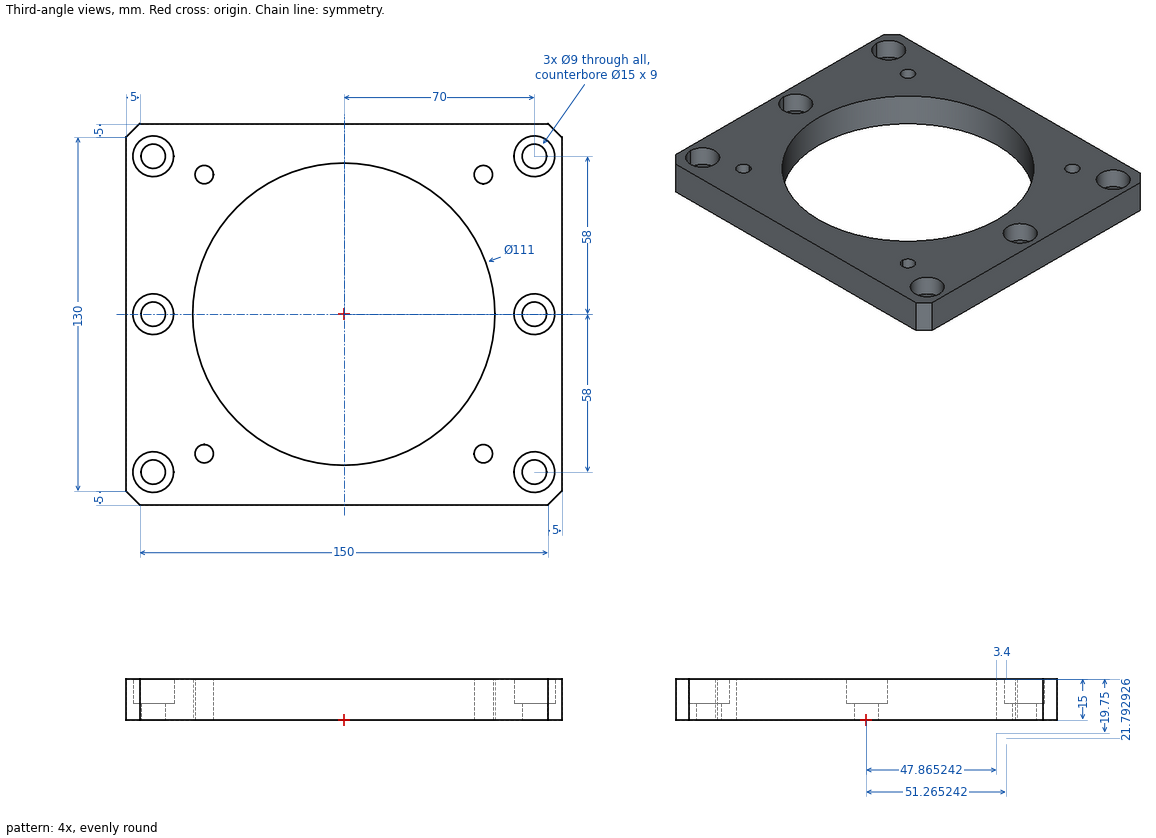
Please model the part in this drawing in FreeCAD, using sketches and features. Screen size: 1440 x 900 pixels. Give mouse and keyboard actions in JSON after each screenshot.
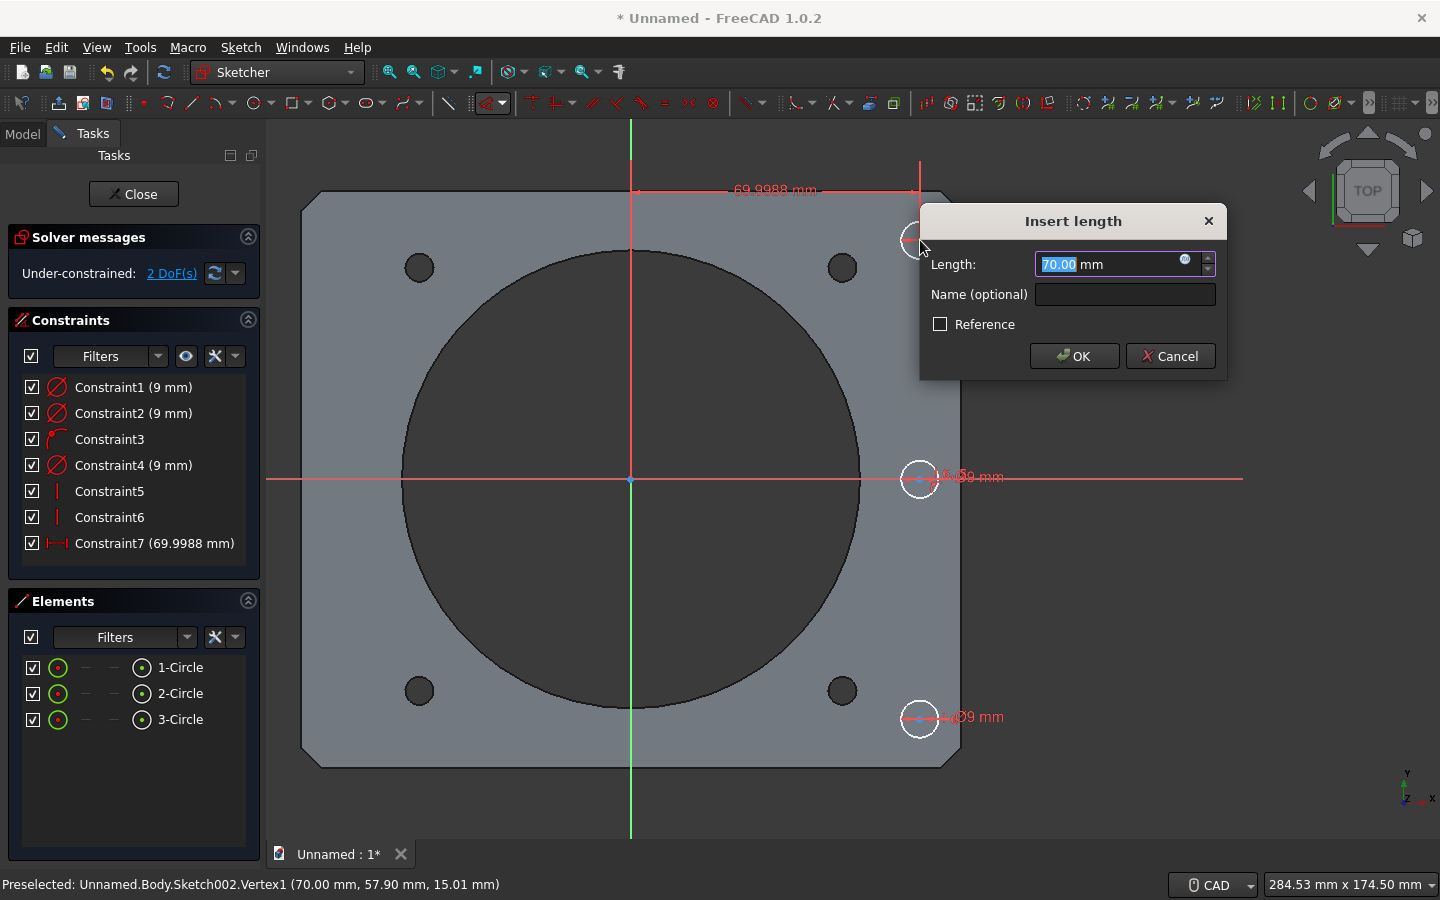
{"action": "type", "text": "70"}
{"action": "key", "text": "Return"}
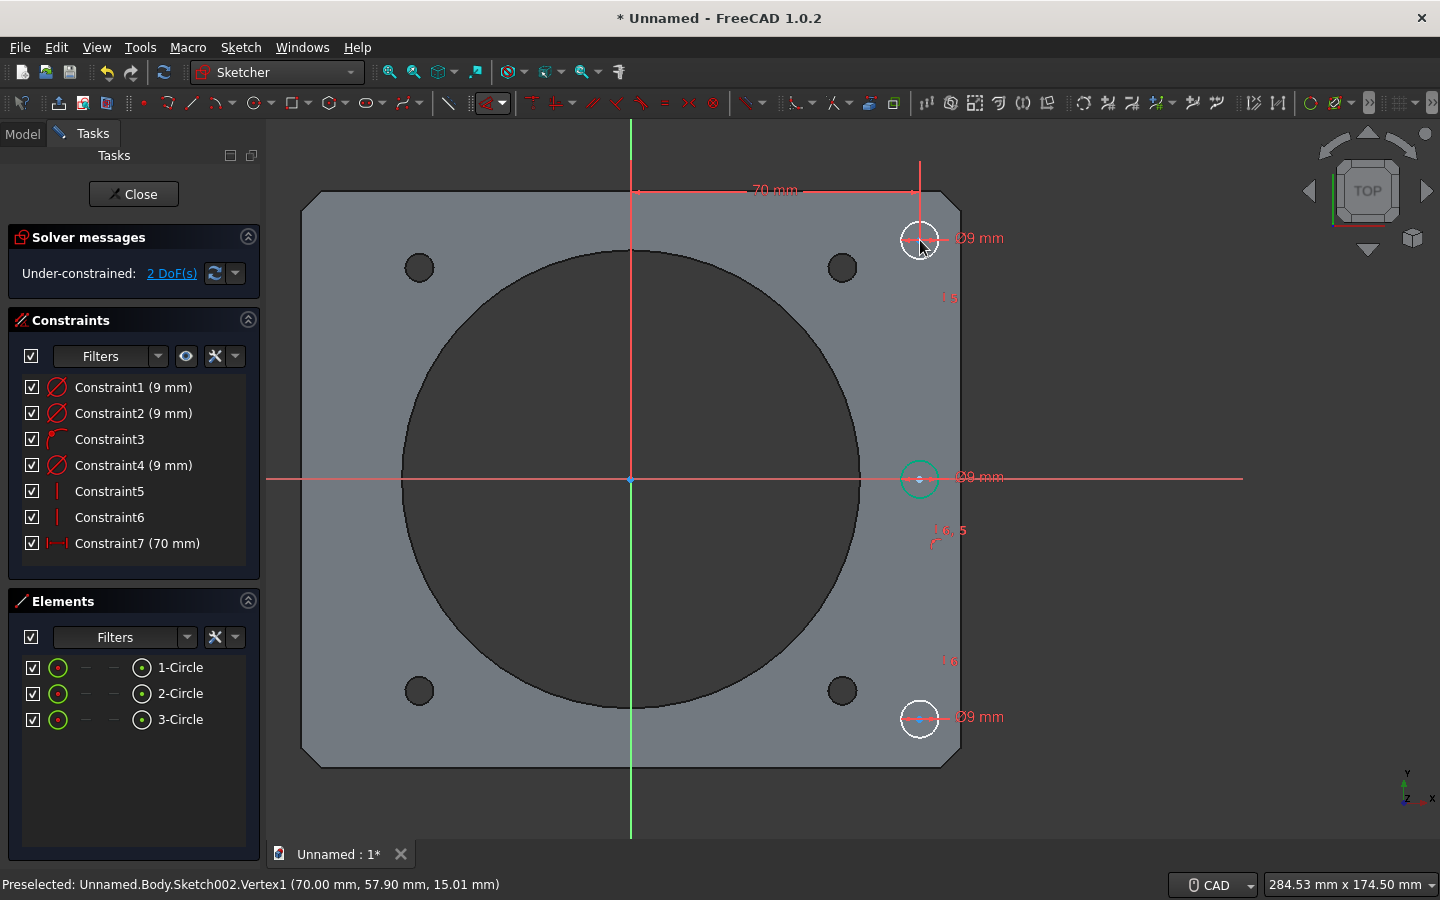
{"action": "left_click", "coordinate": [920, 240]}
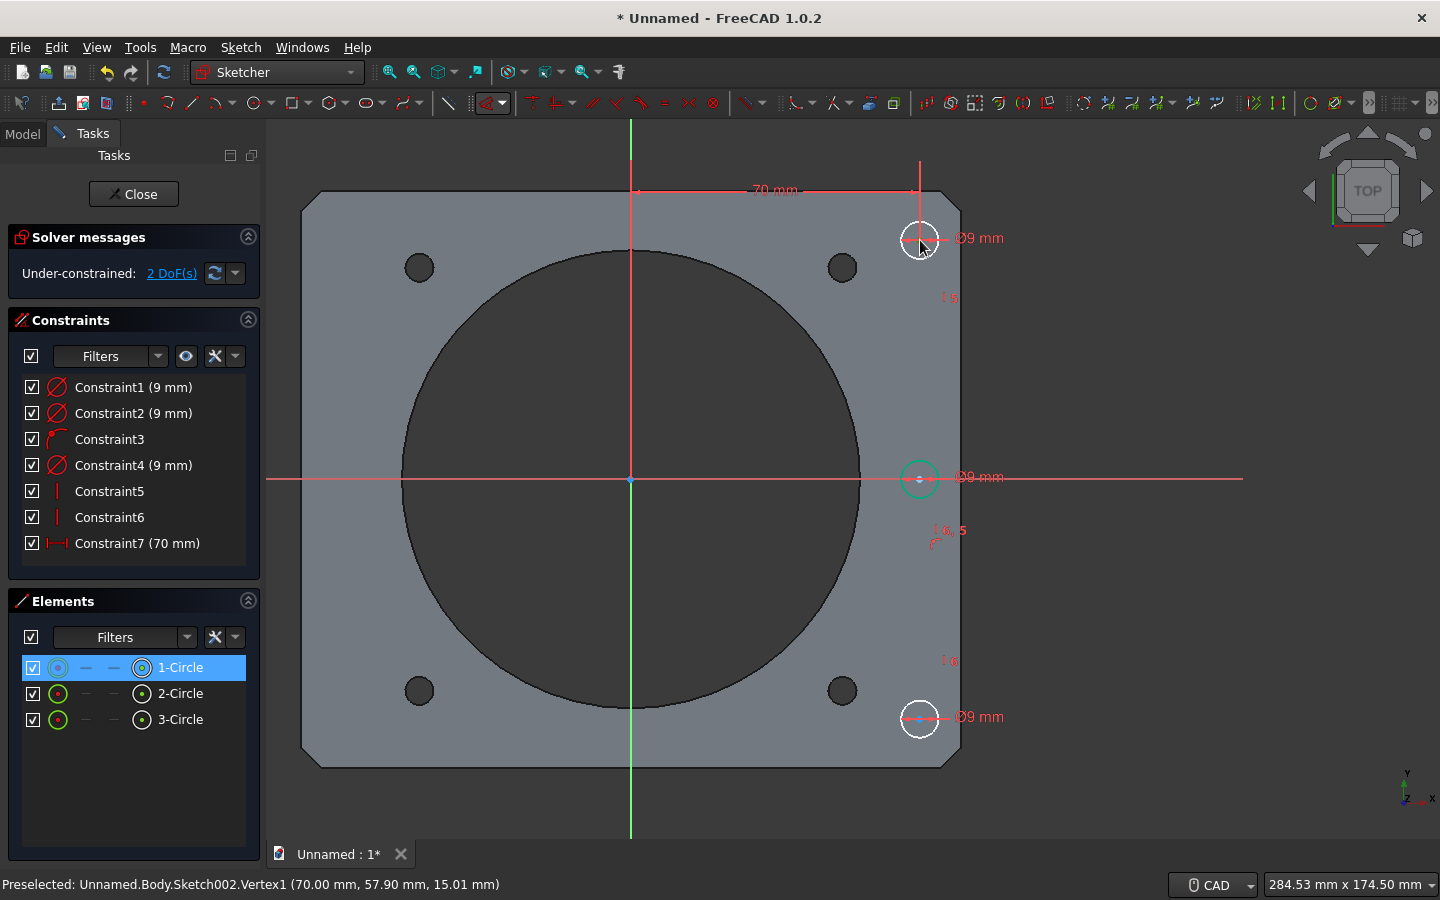
{"action": "left_click", "coordinate": [504, 104]}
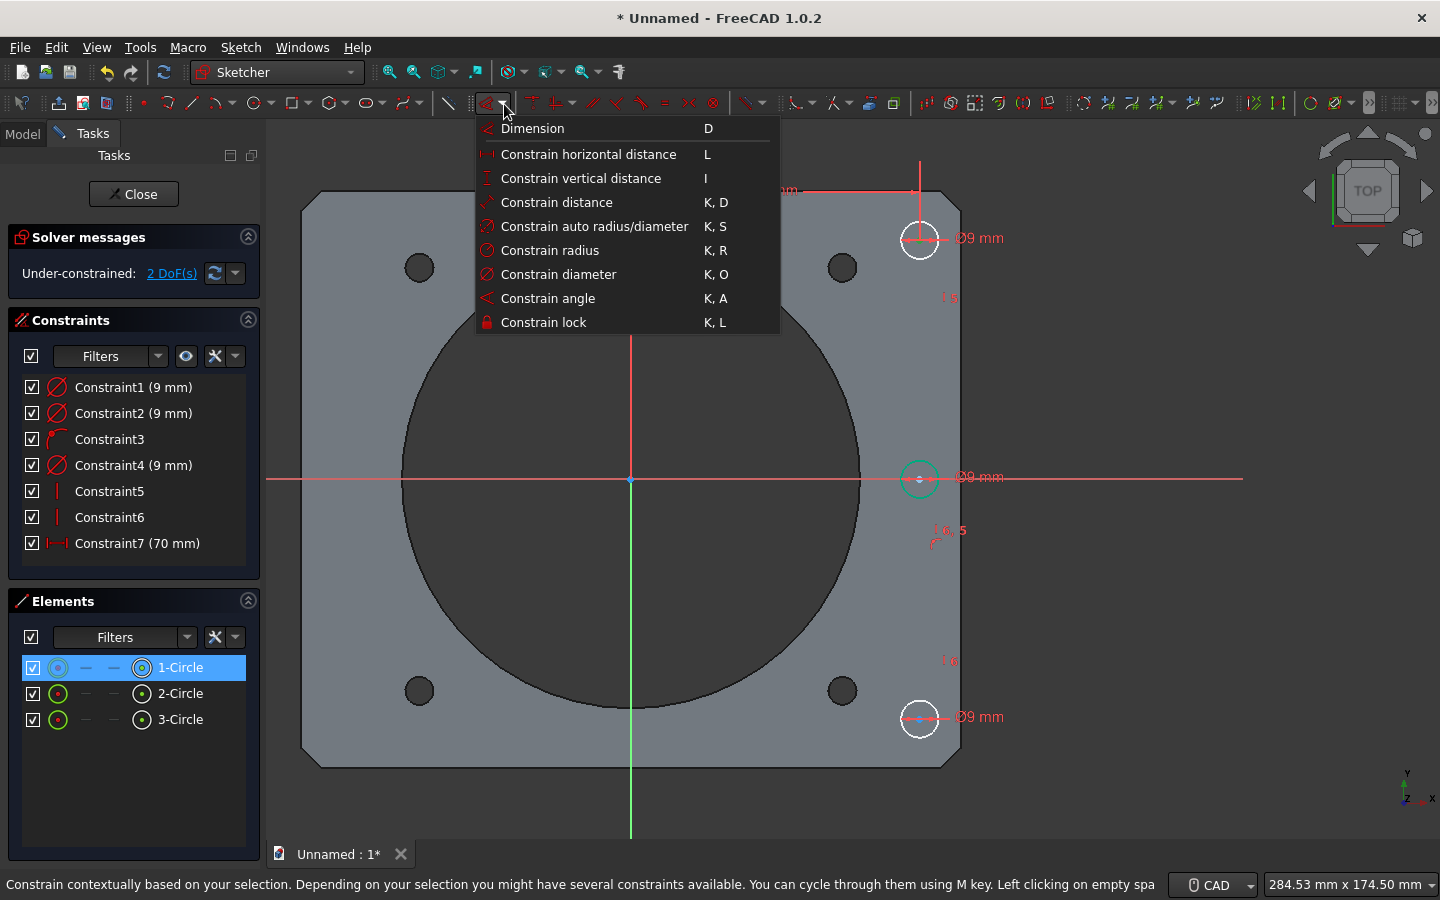
{"action": "left_click", "coordinate": [628, 178]}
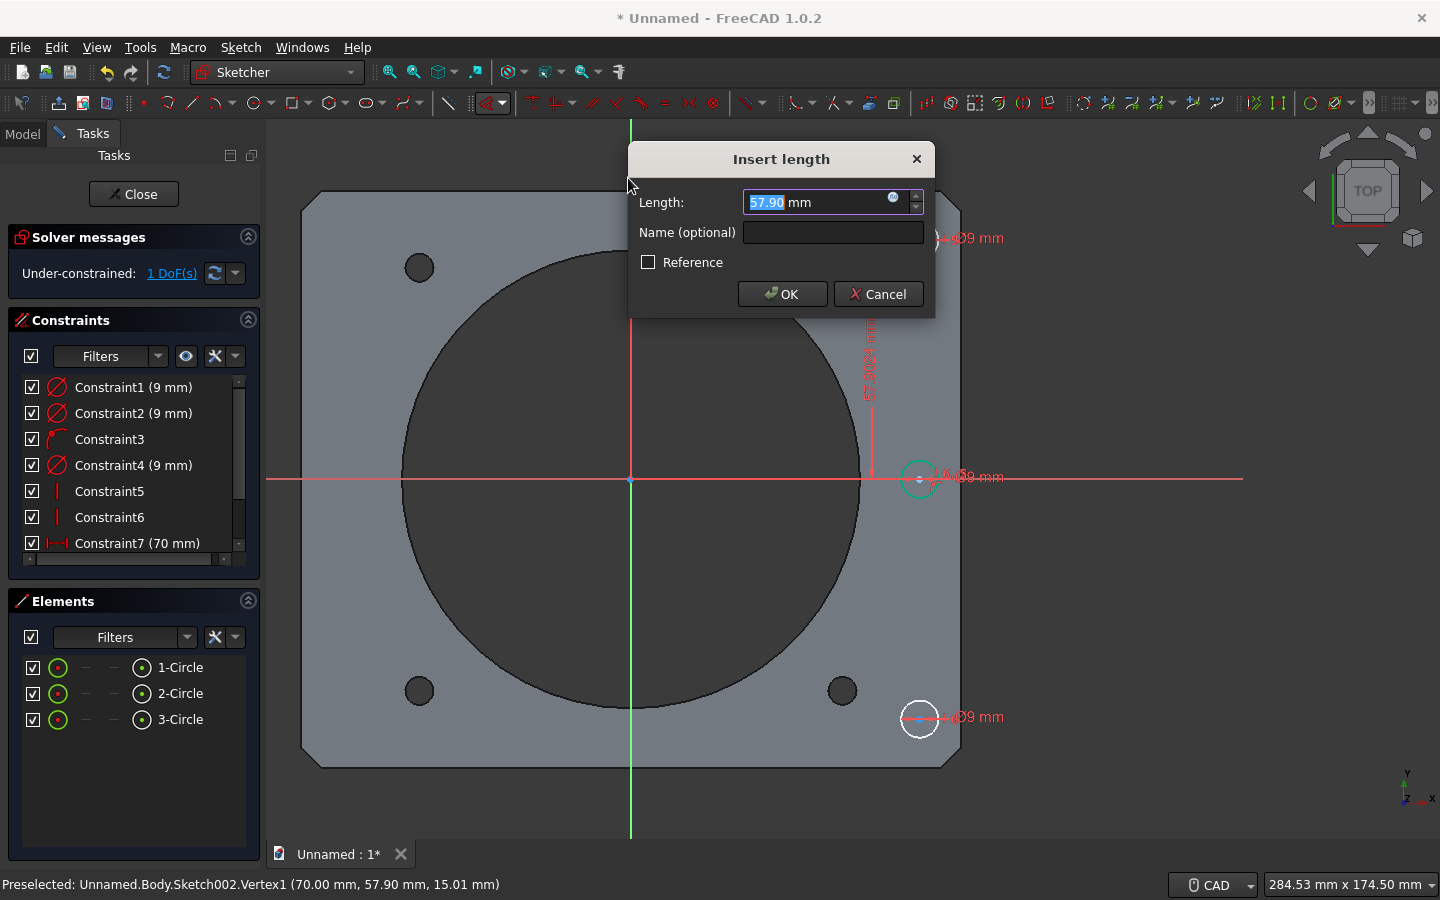
{"action": "type", "text": "58"}
{"action": "key", "text": "Return"}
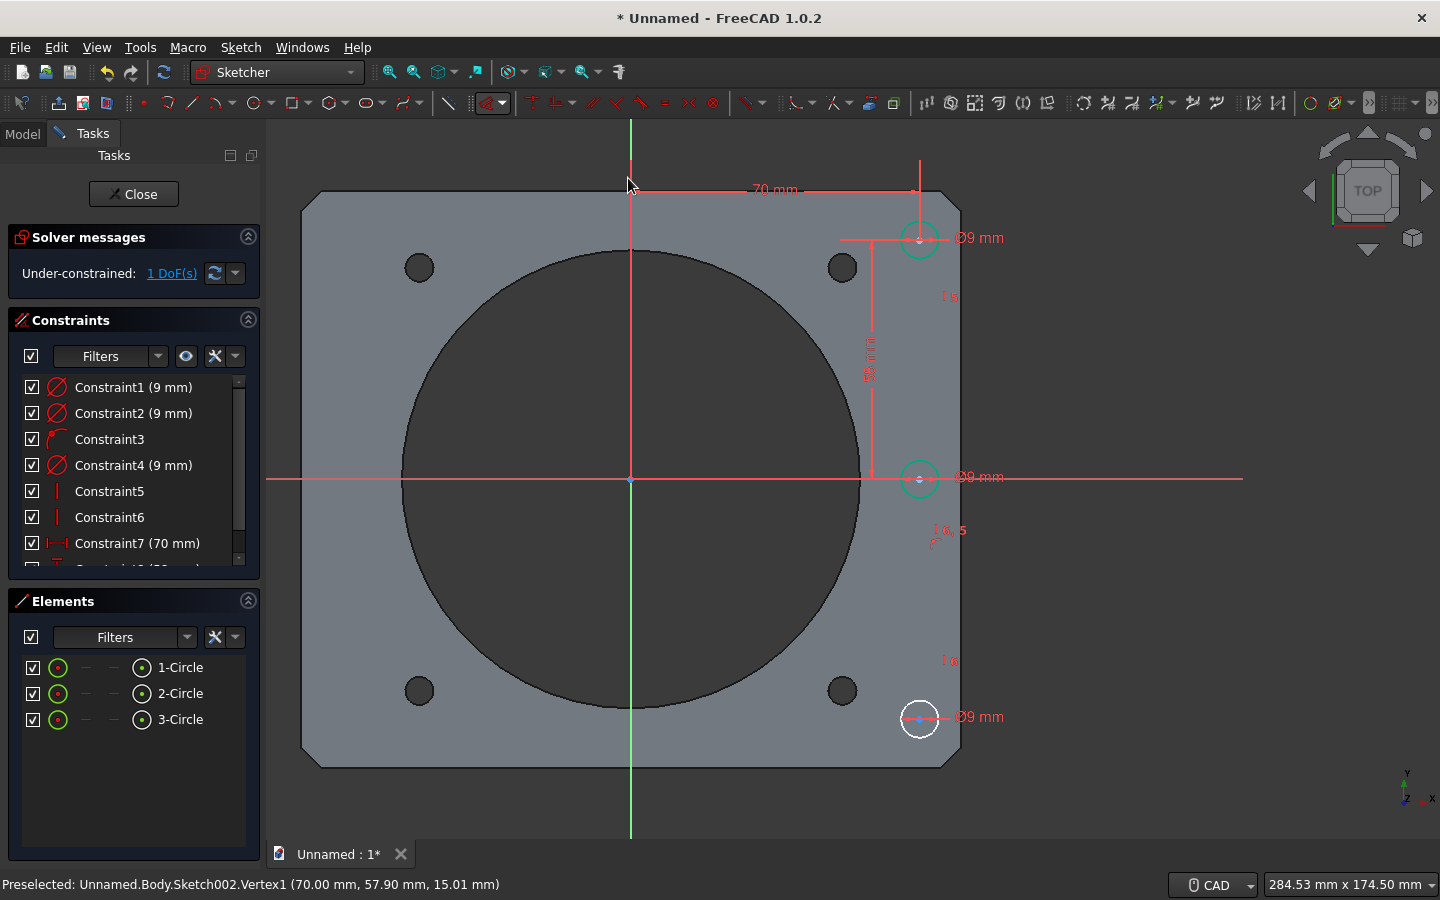
{"action": "left_click", "coordinate": [920, 719]}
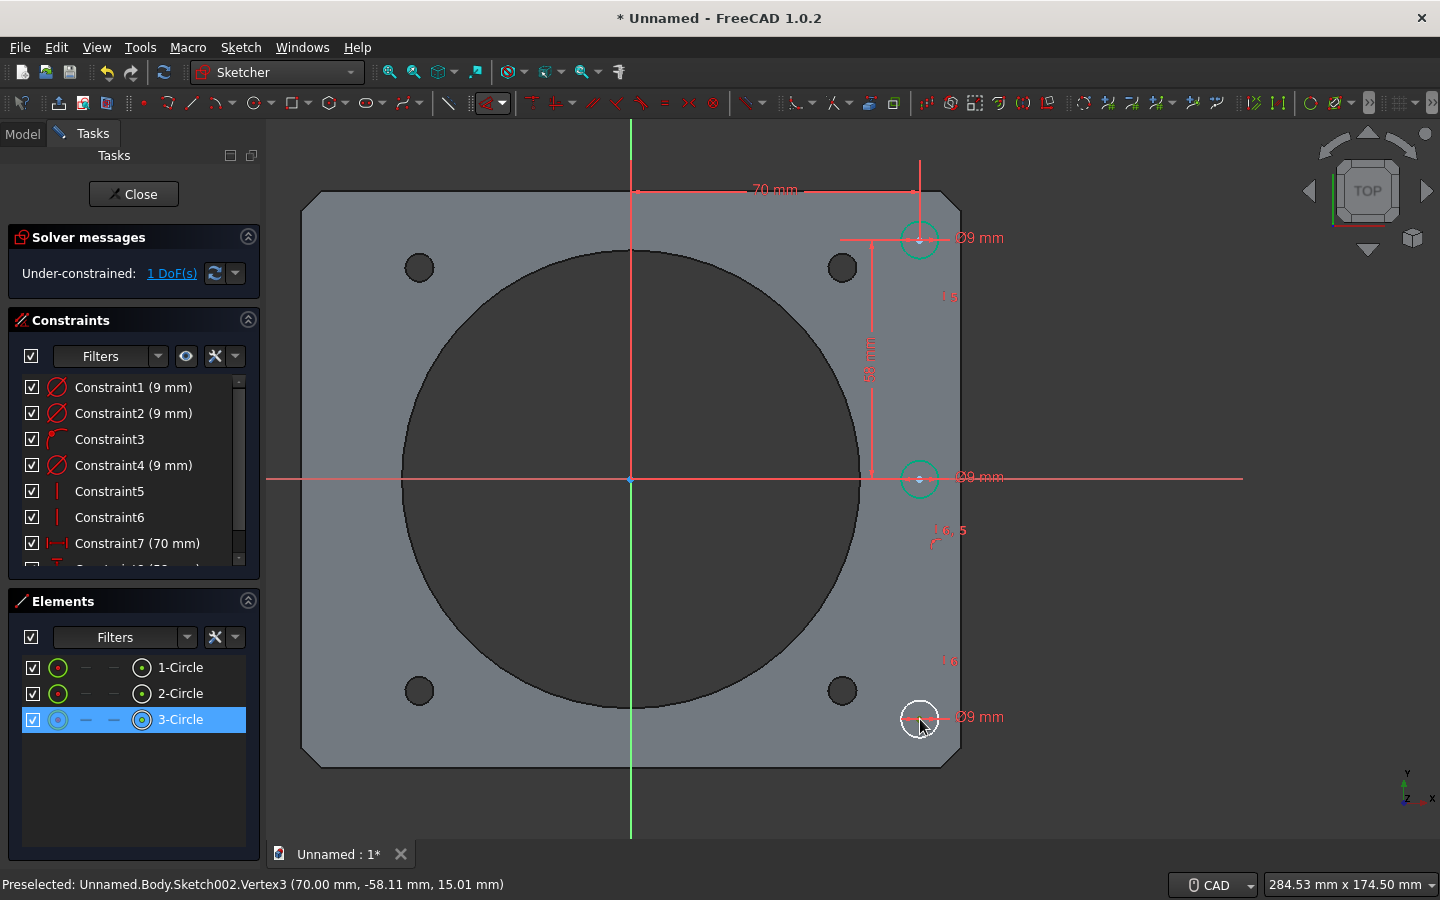
{"action": "key", "text": "i"}